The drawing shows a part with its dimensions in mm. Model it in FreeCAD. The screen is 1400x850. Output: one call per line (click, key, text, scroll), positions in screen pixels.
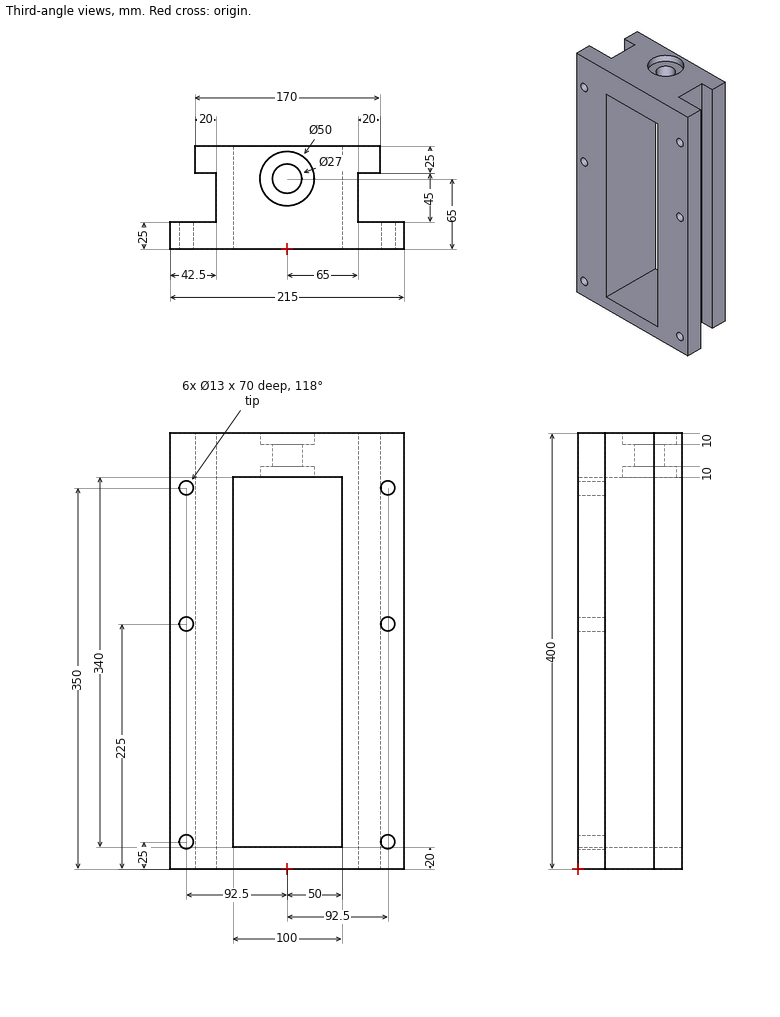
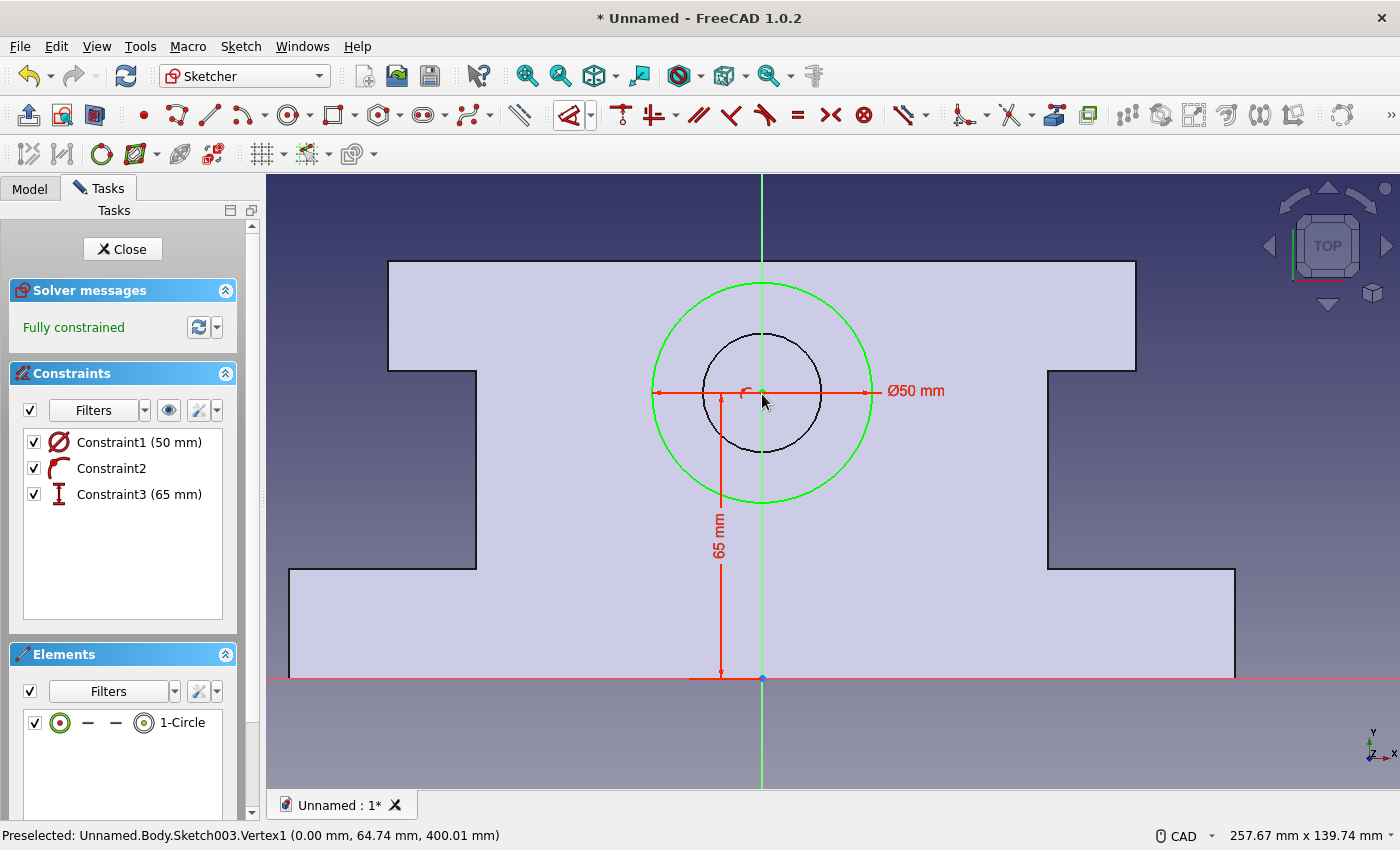
click(123, 249)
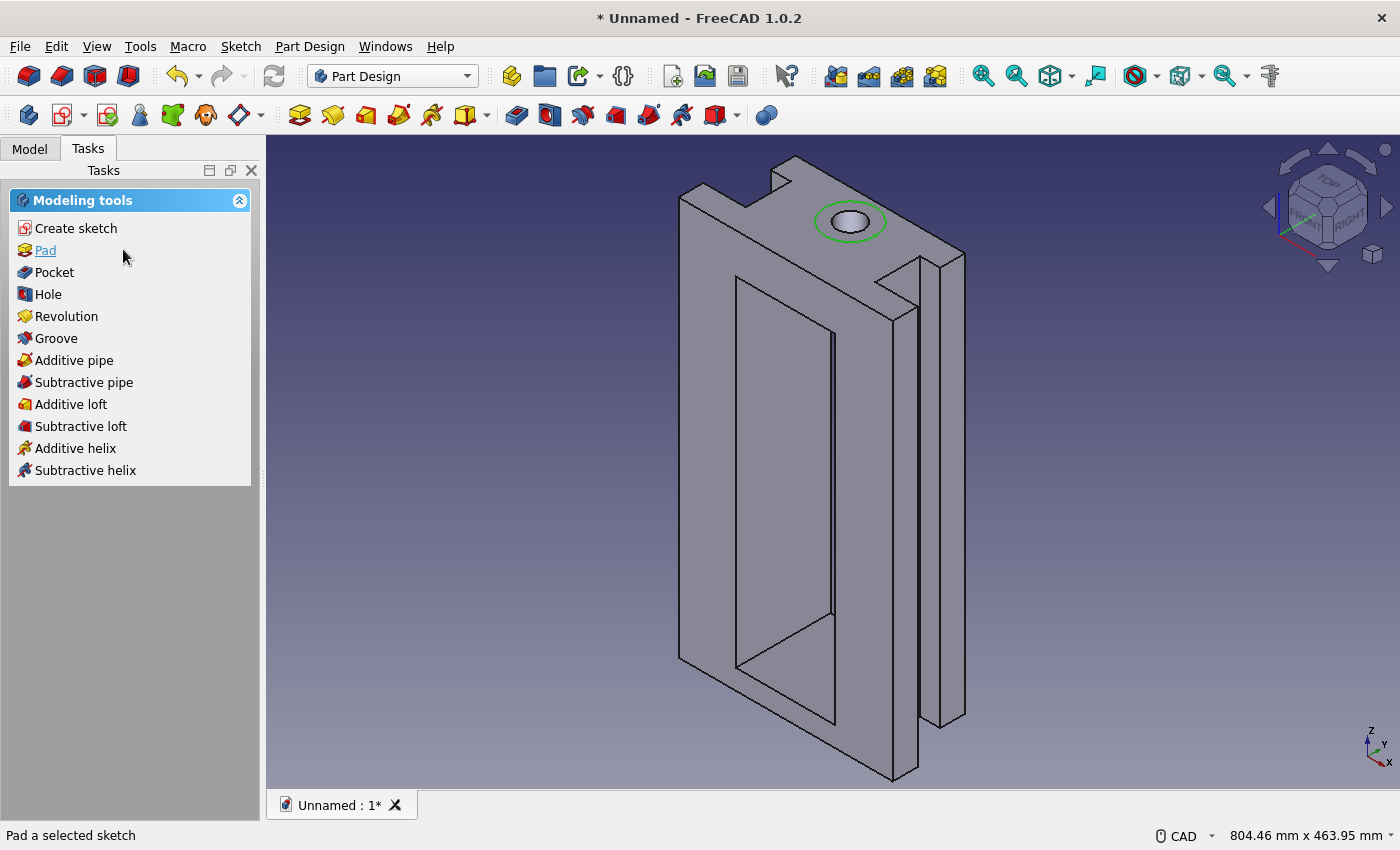
click(517, 116)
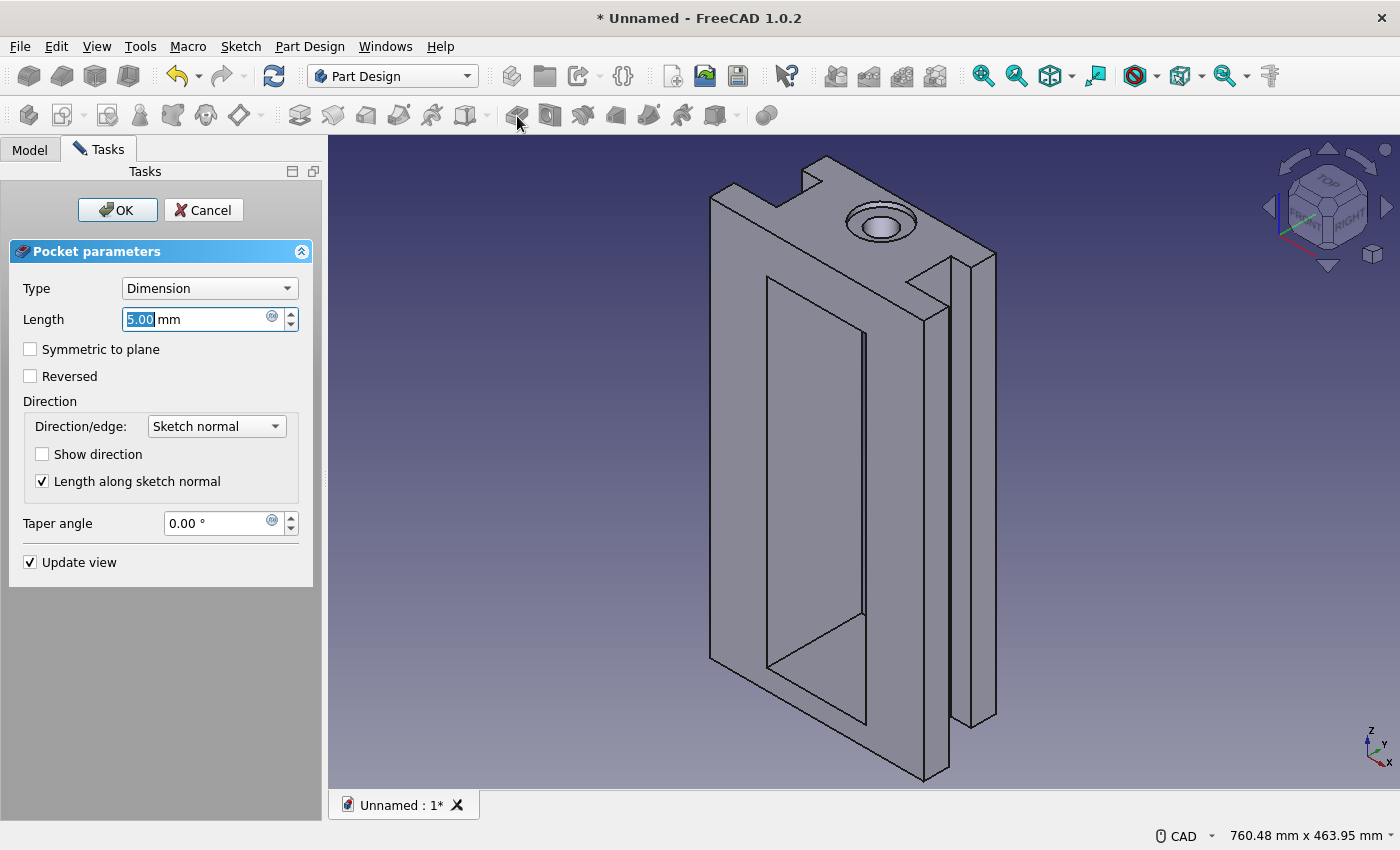
text(10)
key(Tab)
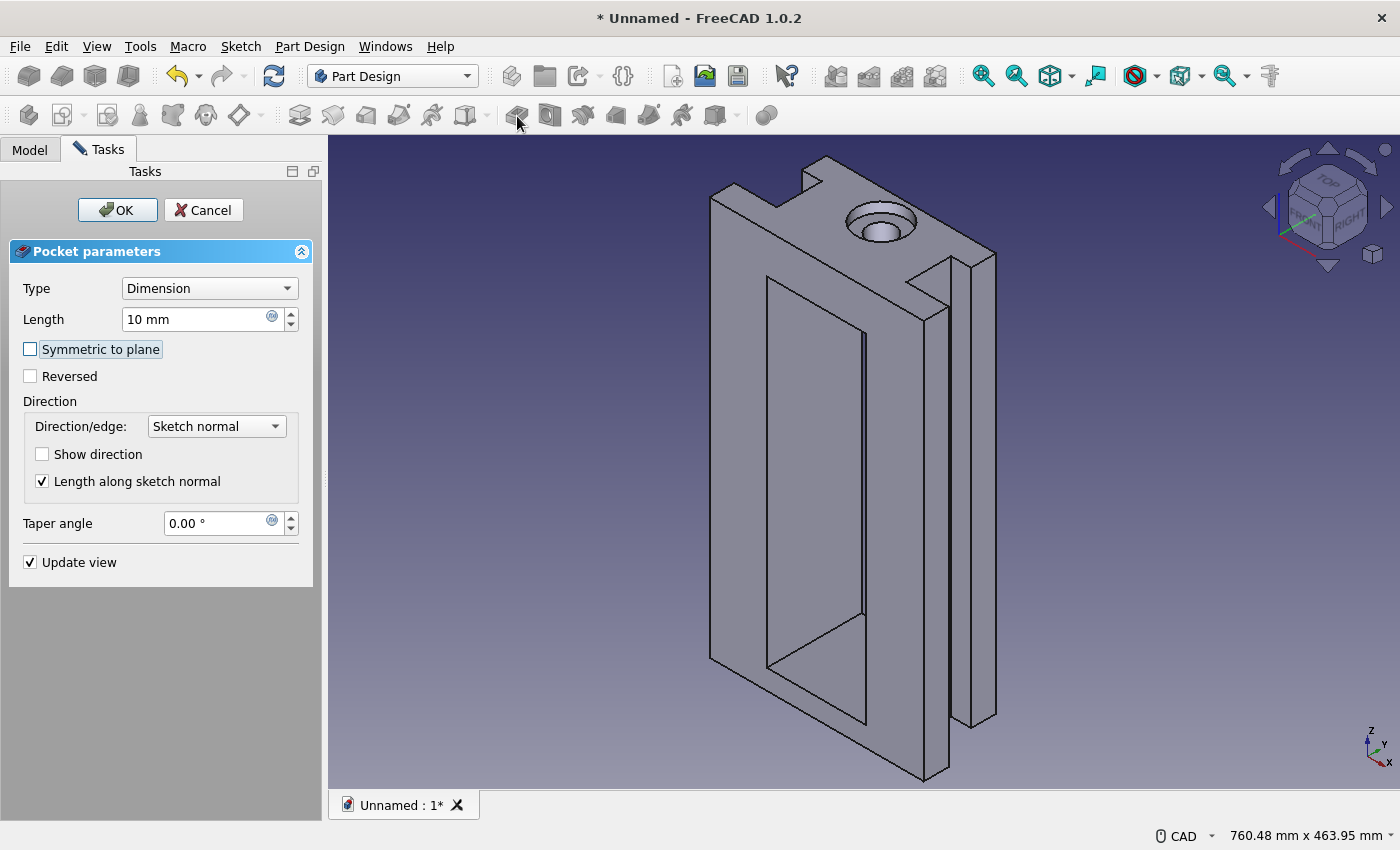
click(118, 210)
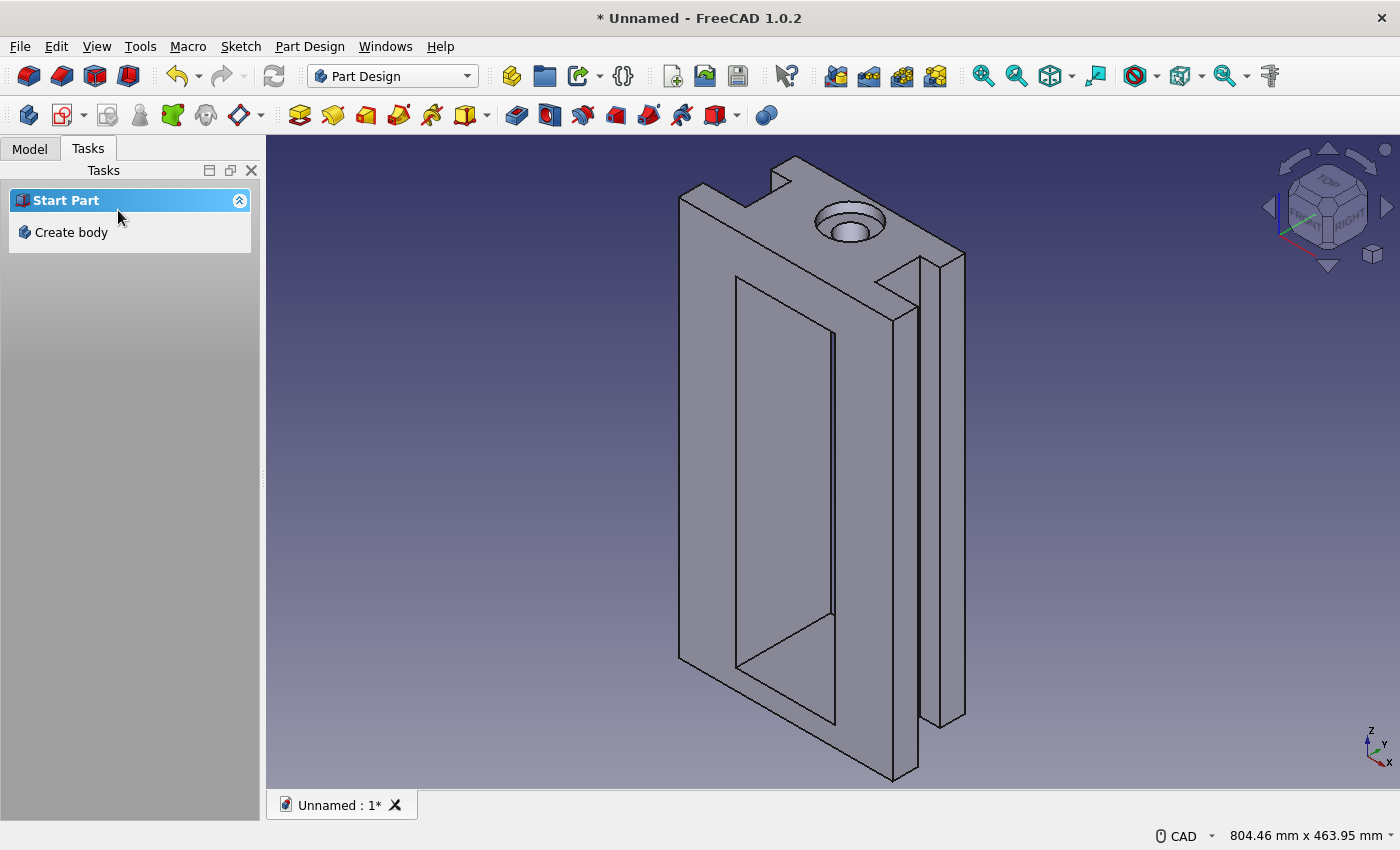
click(30, 148)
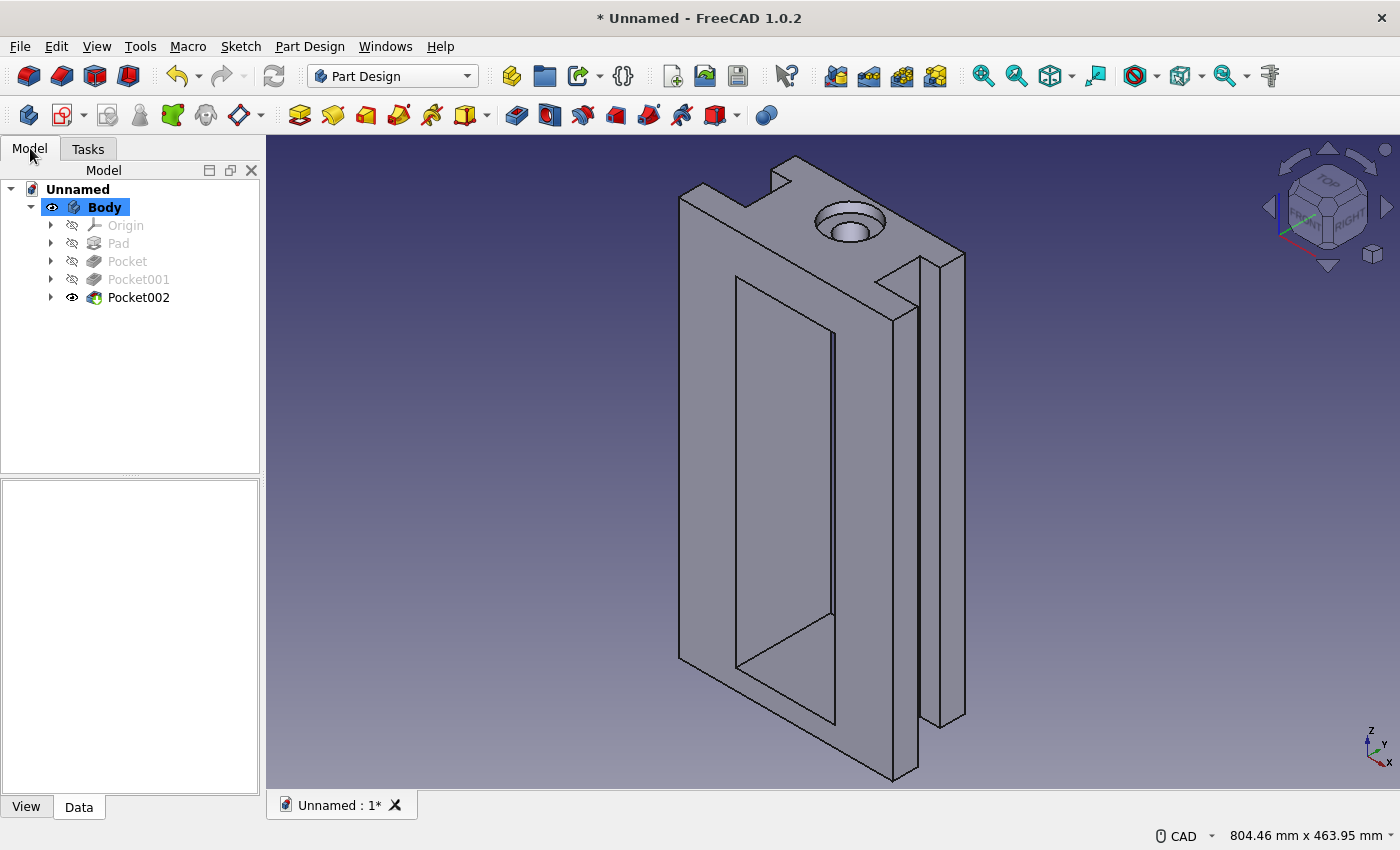
click(51, 225)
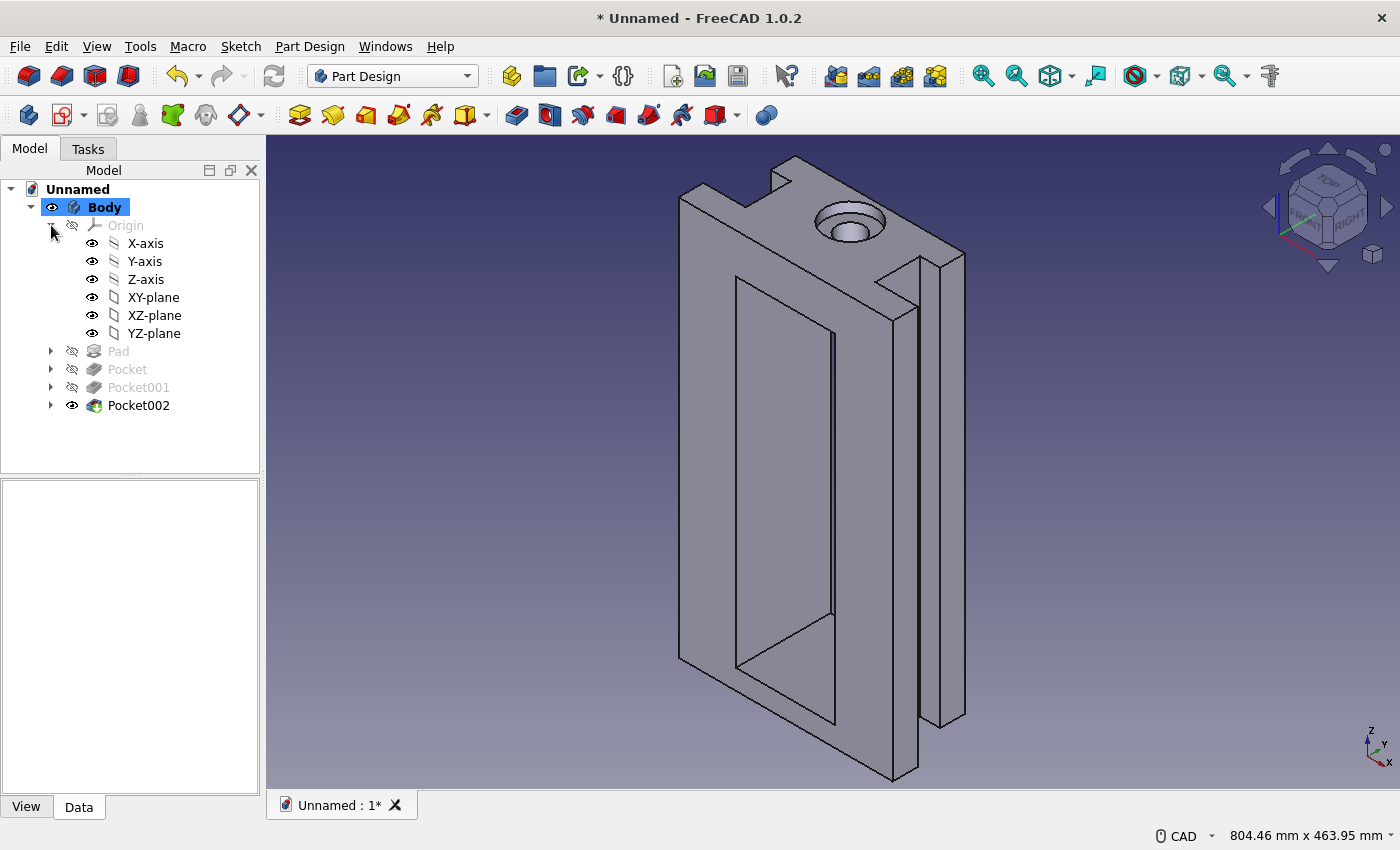
click(137, 297)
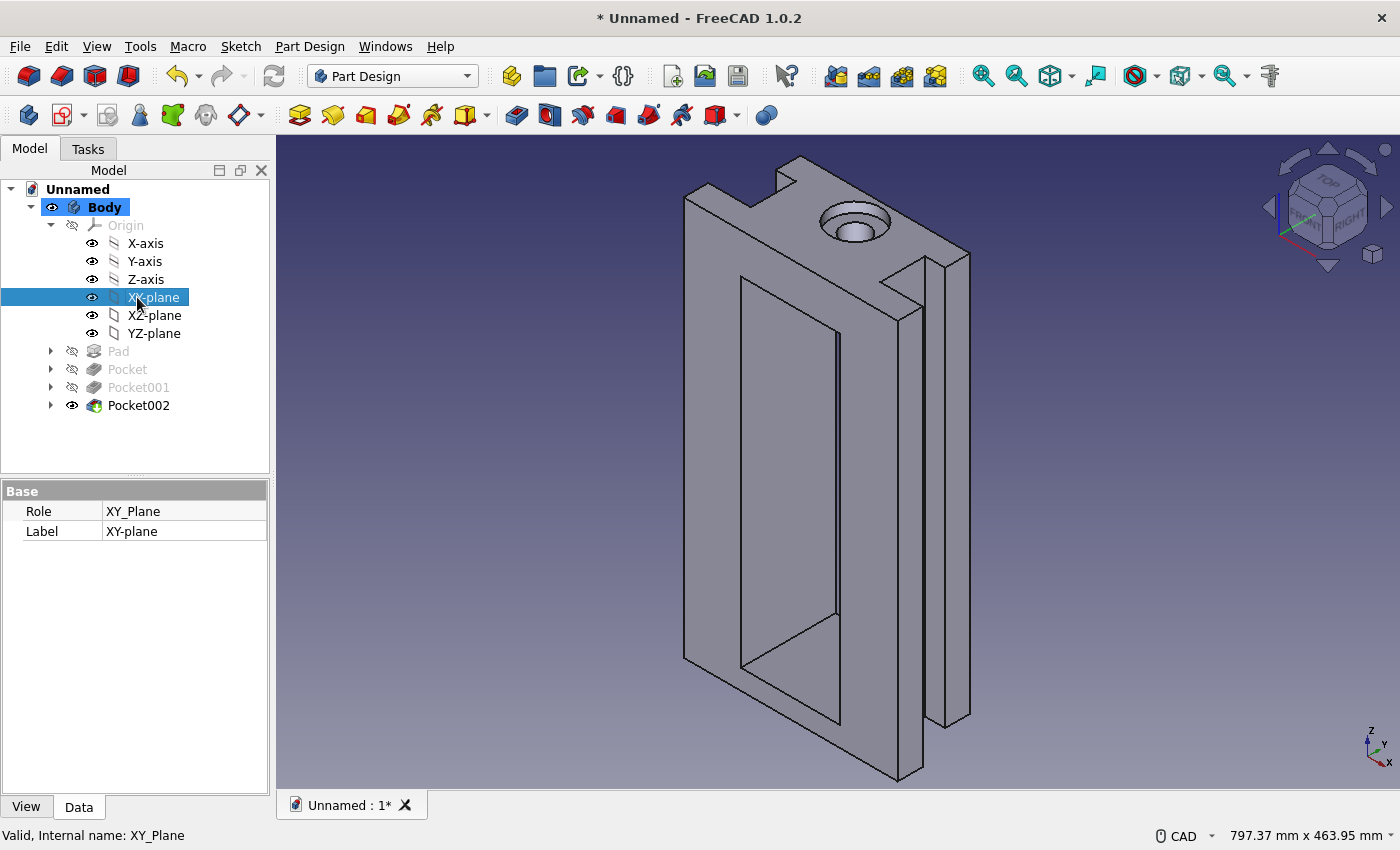
click(238, 116)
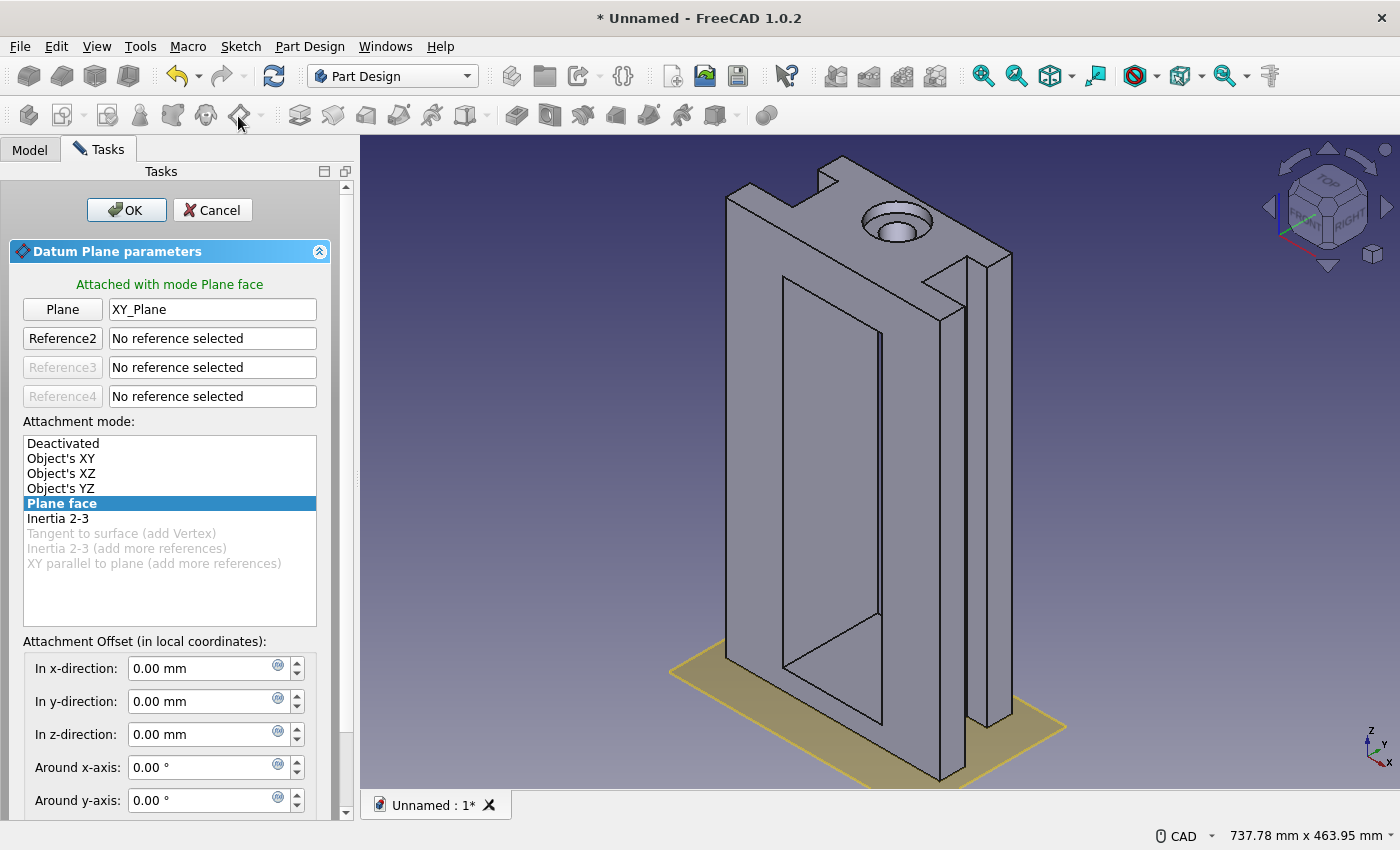
triple_click(210, 734)